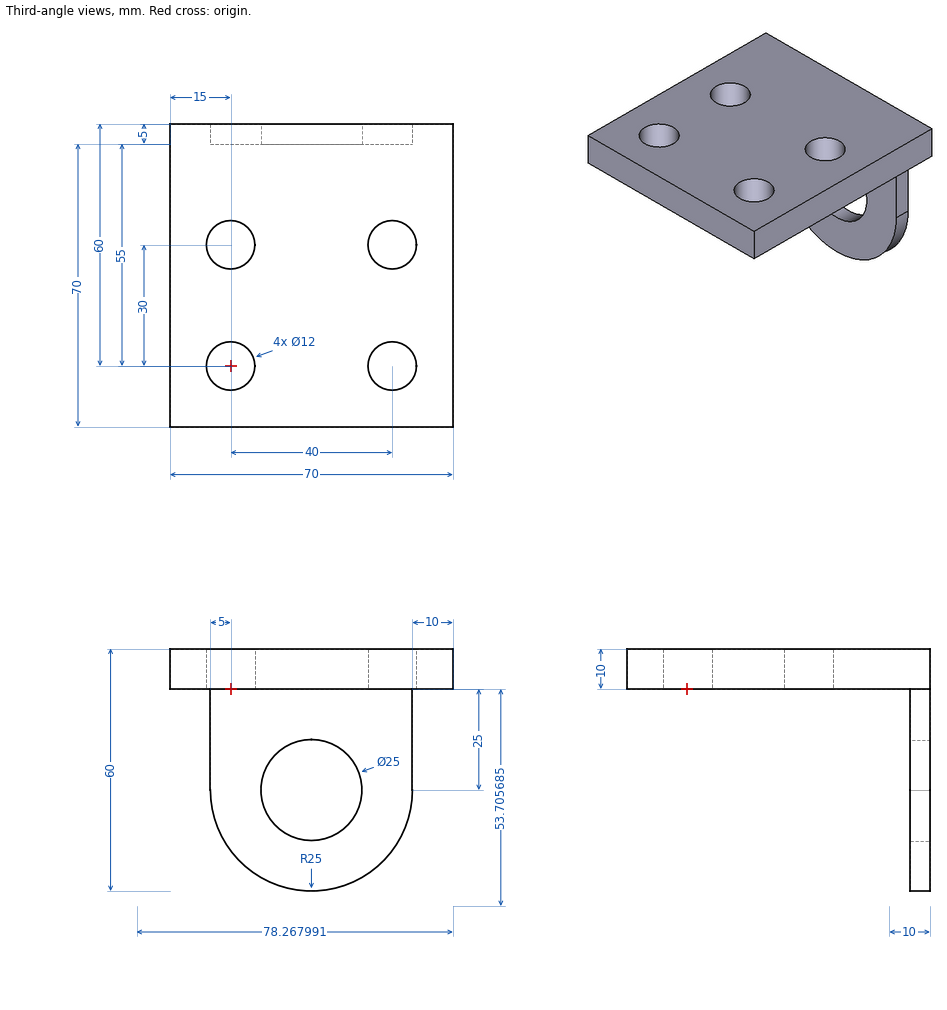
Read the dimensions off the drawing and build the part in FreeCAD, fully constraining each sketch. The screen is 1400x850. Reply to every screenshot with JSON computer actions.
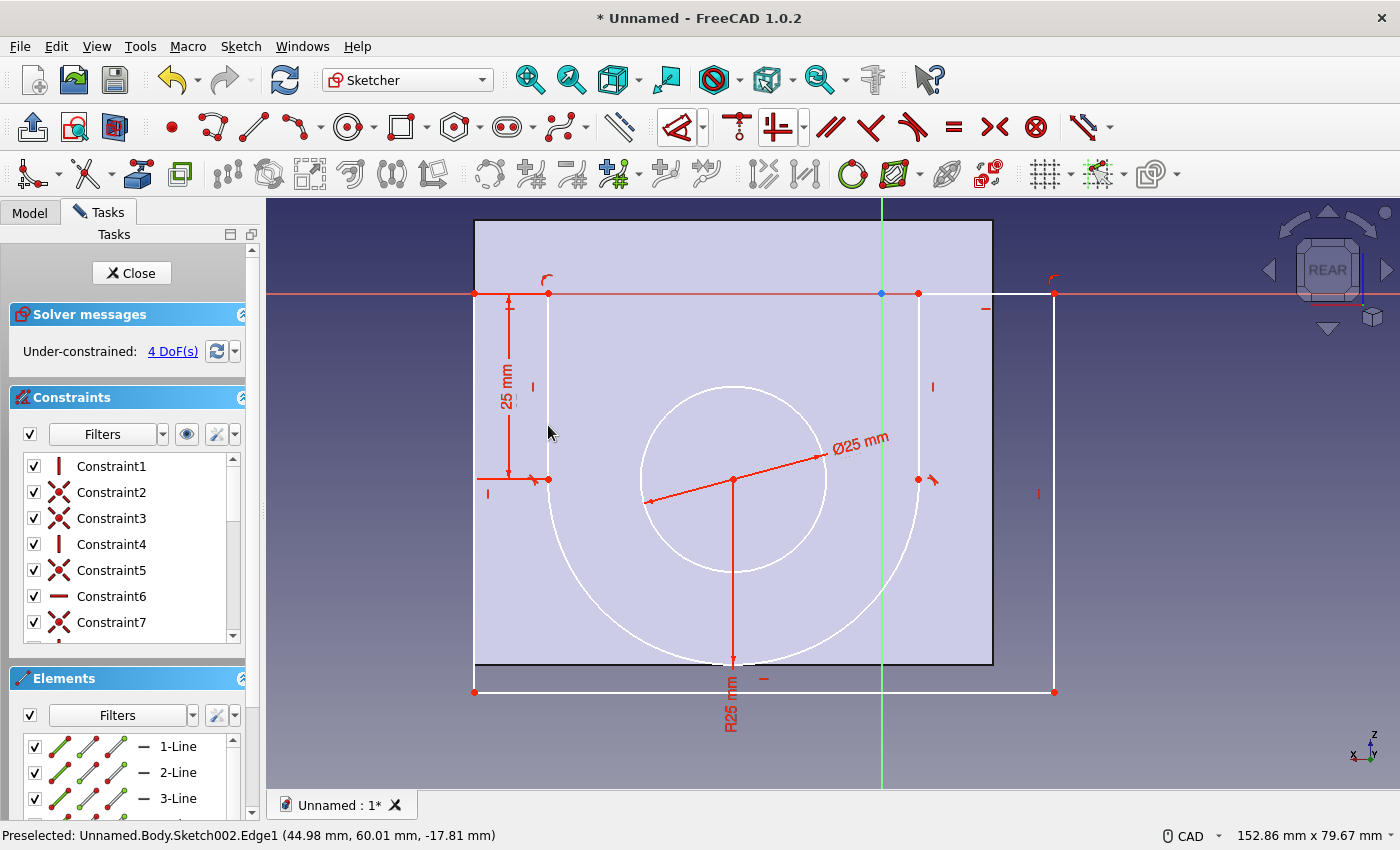
{"action": "left_click", "coordinate": [526, 294]}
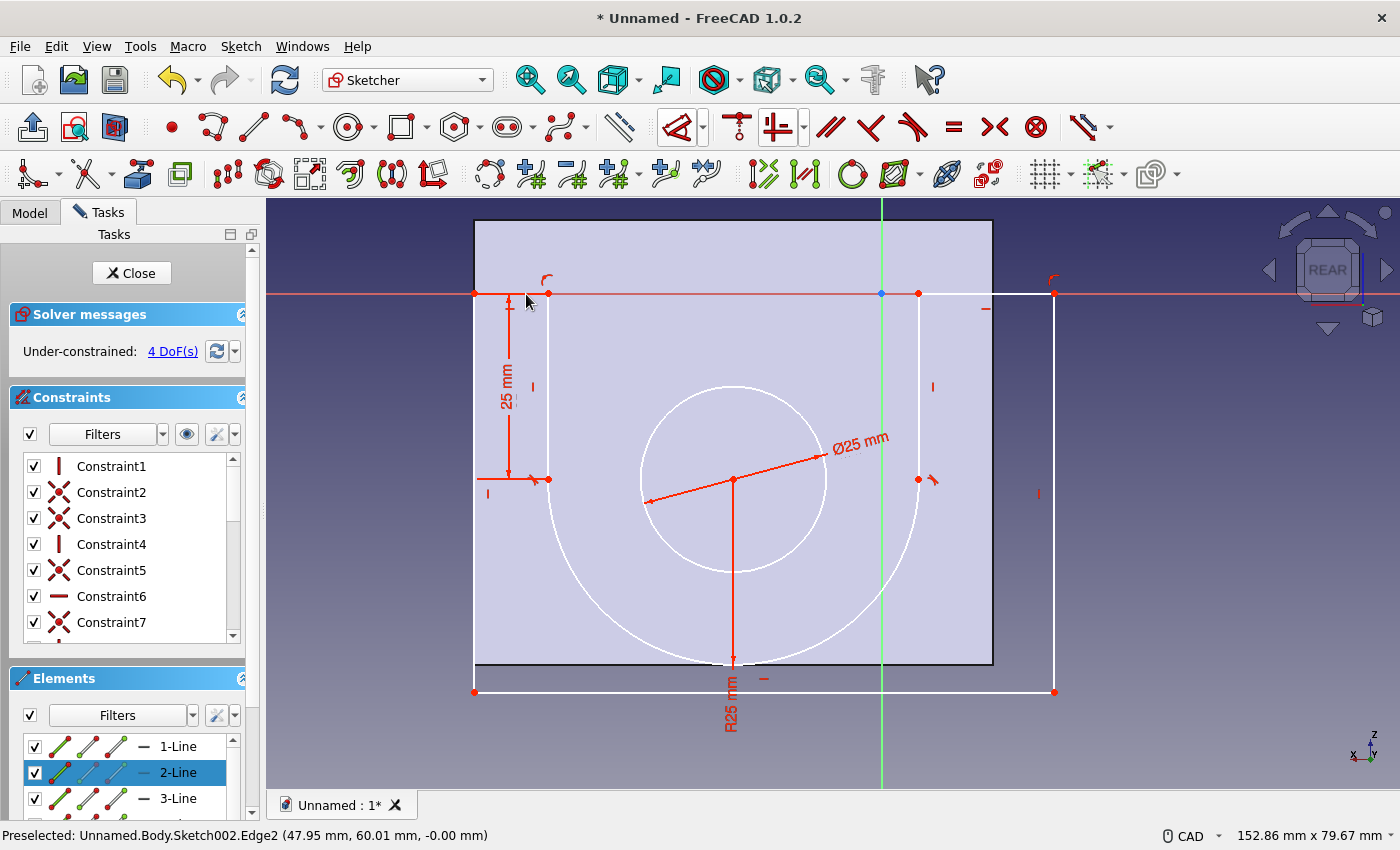
{"action": "left_click", "coordinate": [702, 128]}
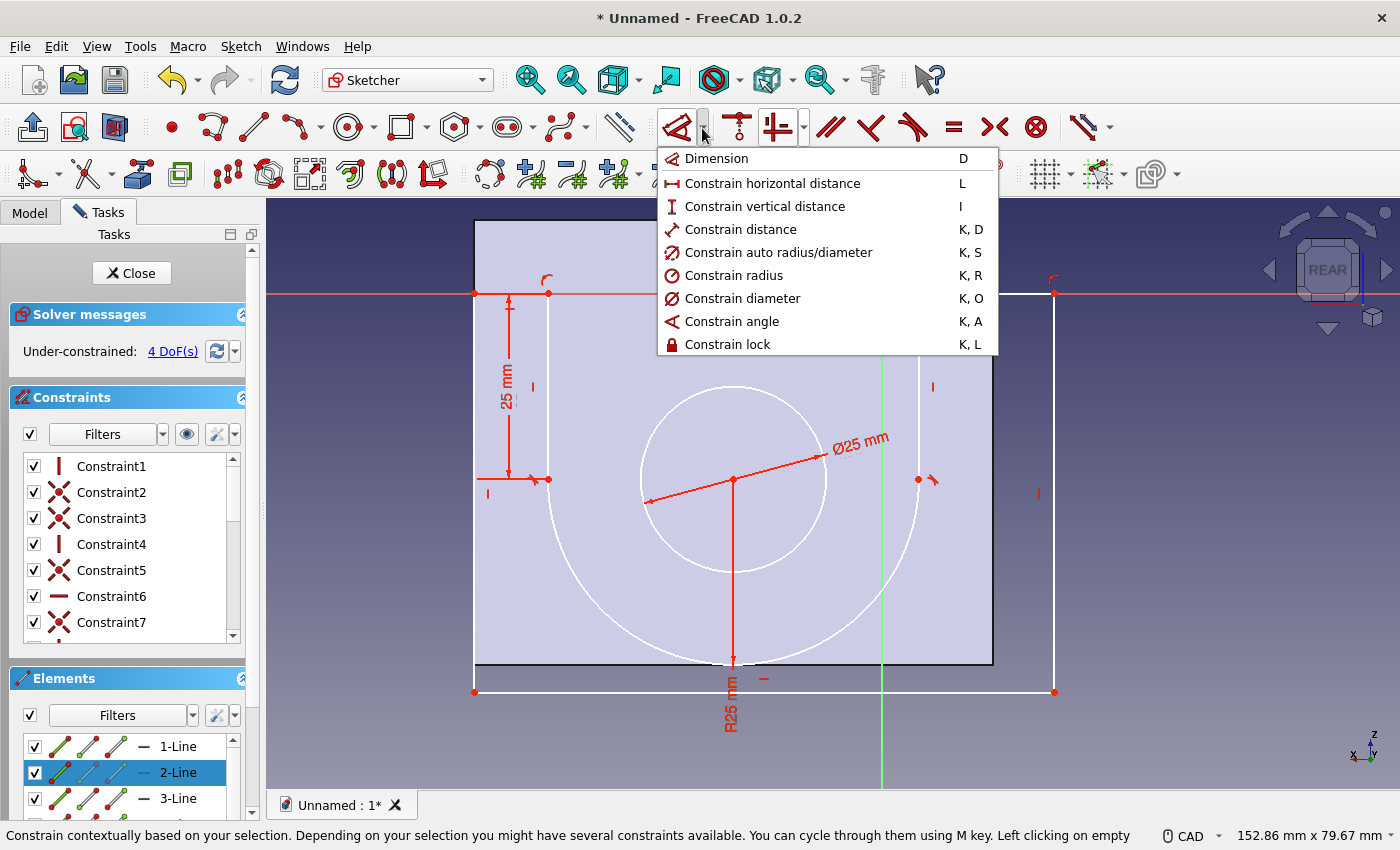
{"action": "left_click", "coordinate": [828, 184]}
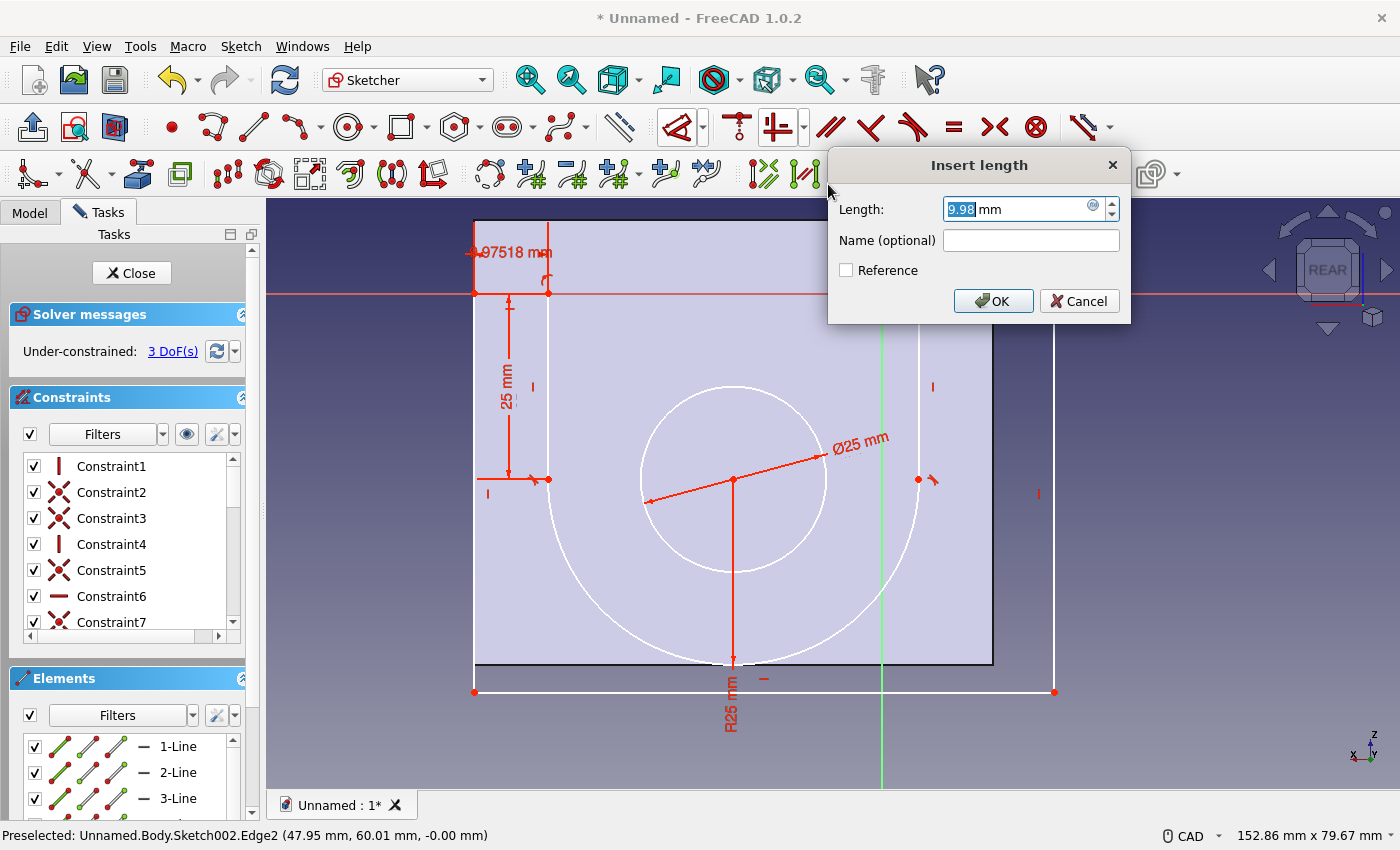
{"action": "type", "text": "10"}
{"action": "key", "text": "Return"}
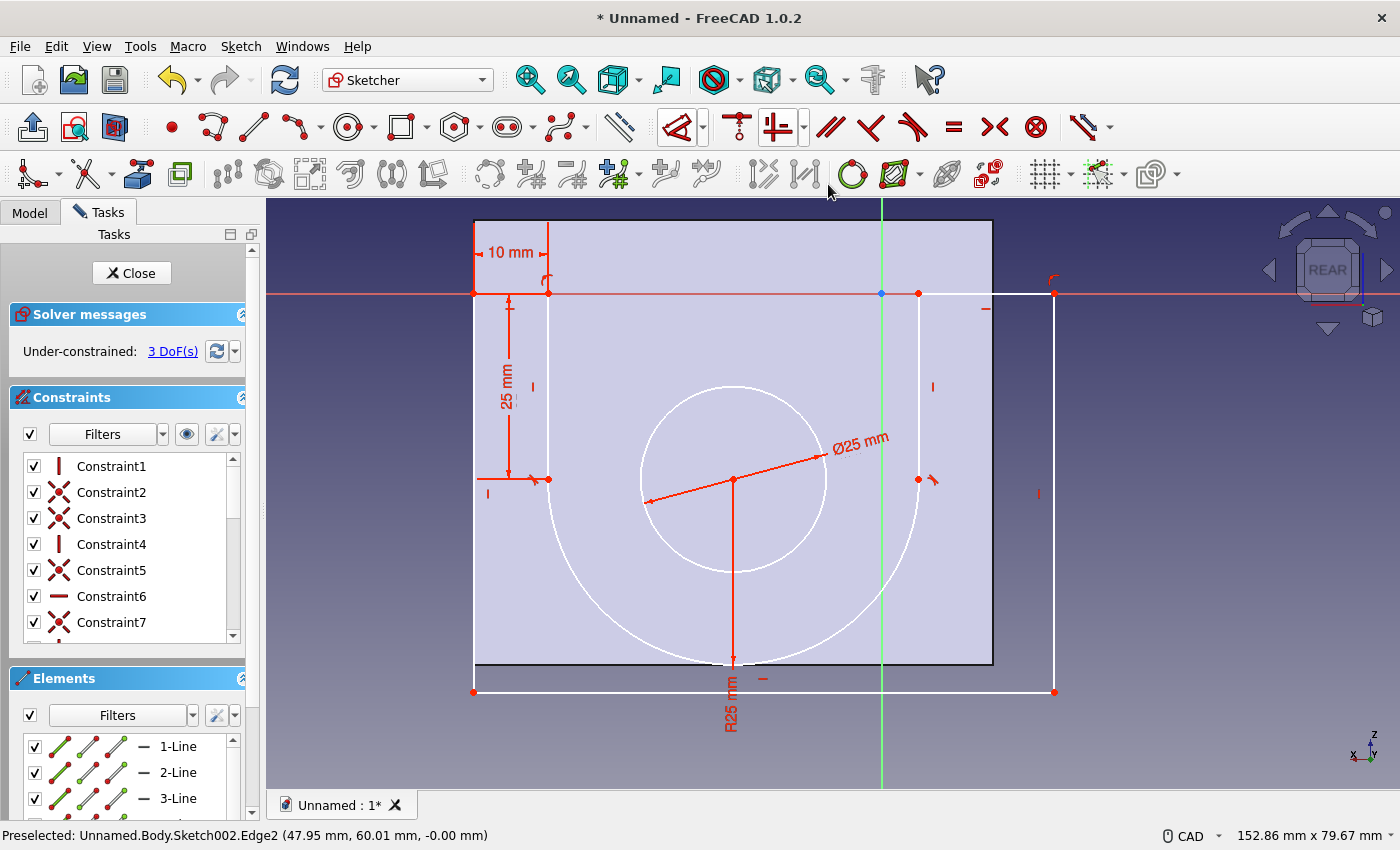
{"action": "left_click", "coordinate": [919, 294]}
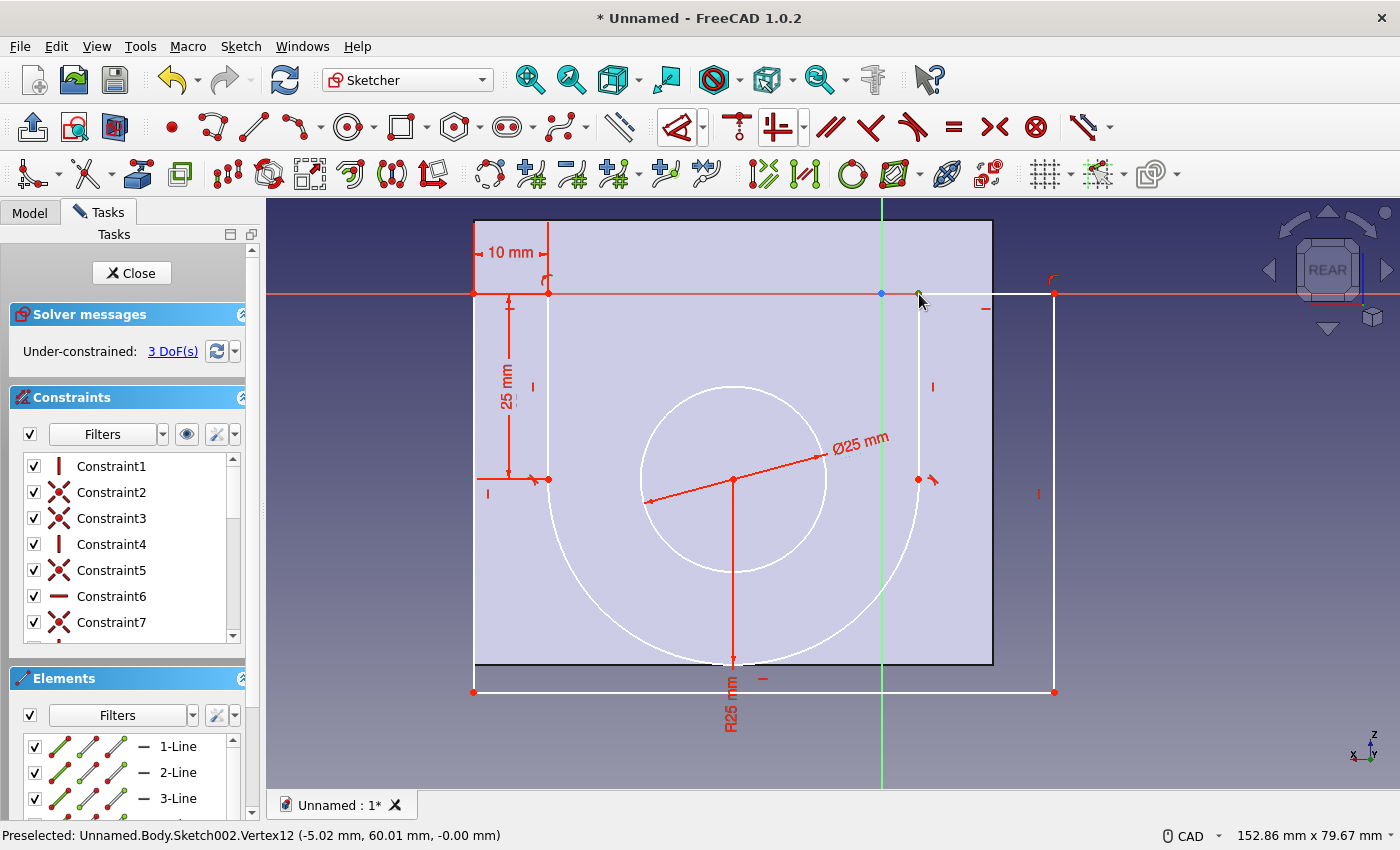
{"action": "left_click", "coordinate": [702, 128]}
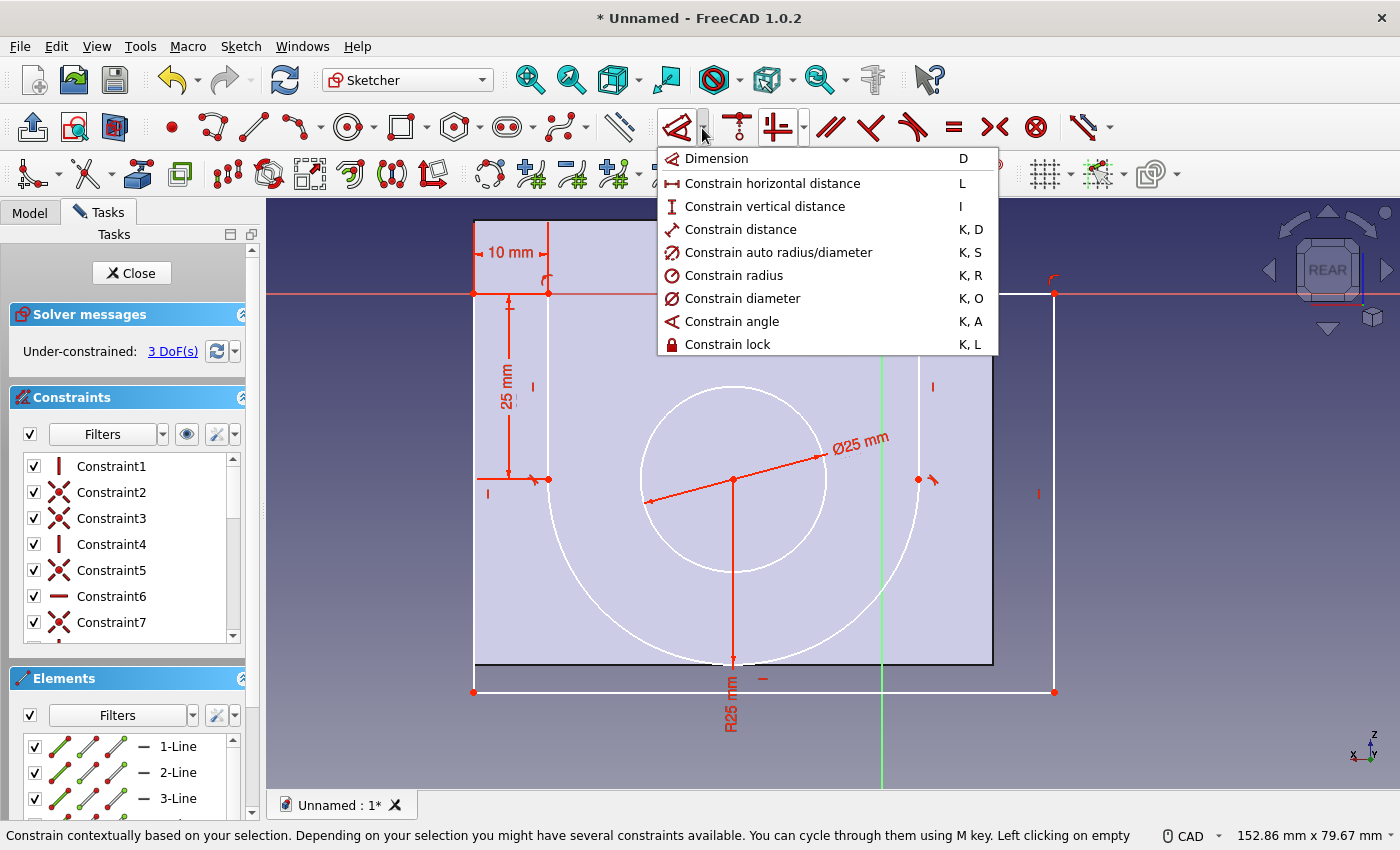
{"action": "left_click", "coordinate": [828, 184]}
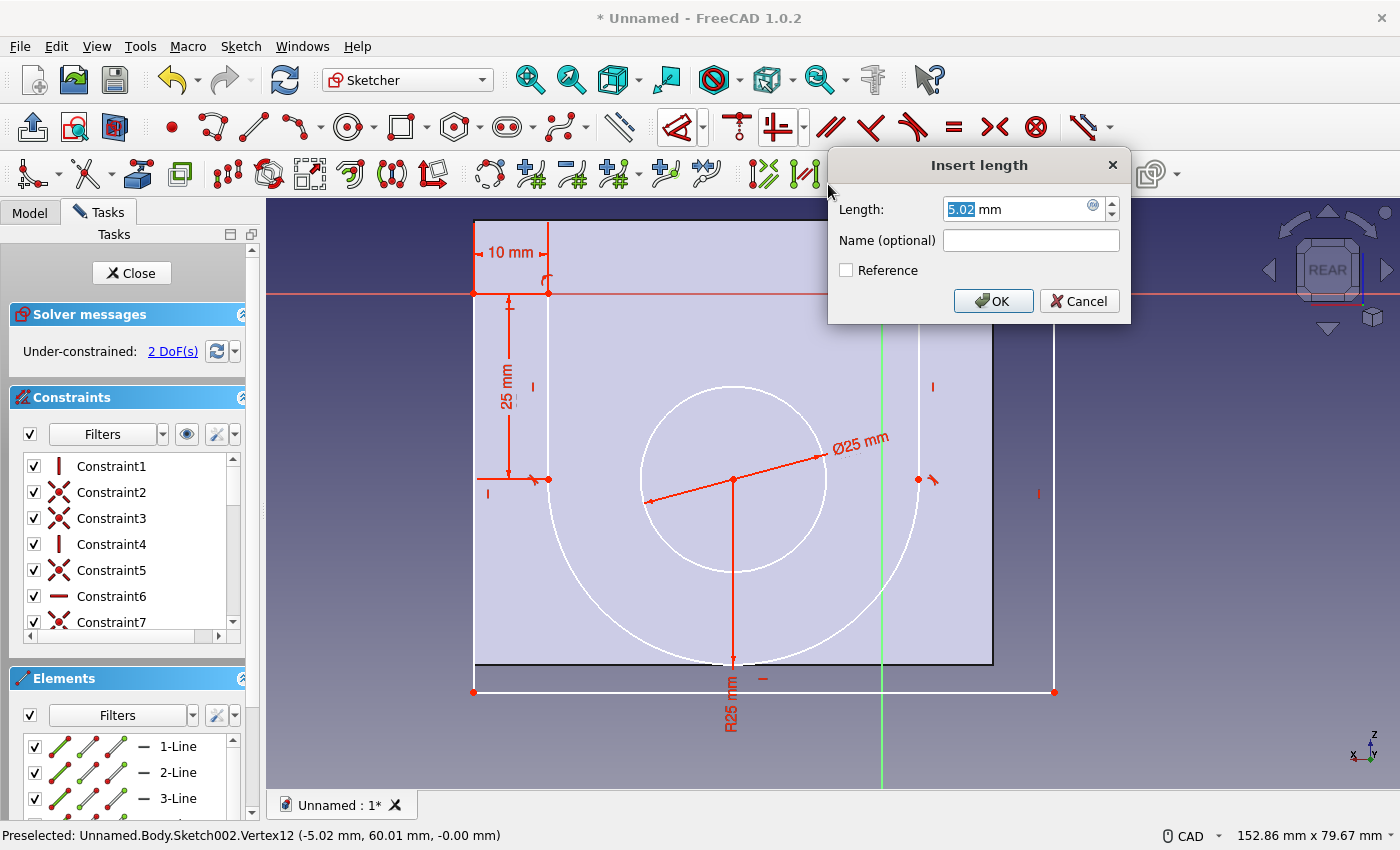
{"action": "type", "text": "5"}
{"action": "key", "text": "Return"}